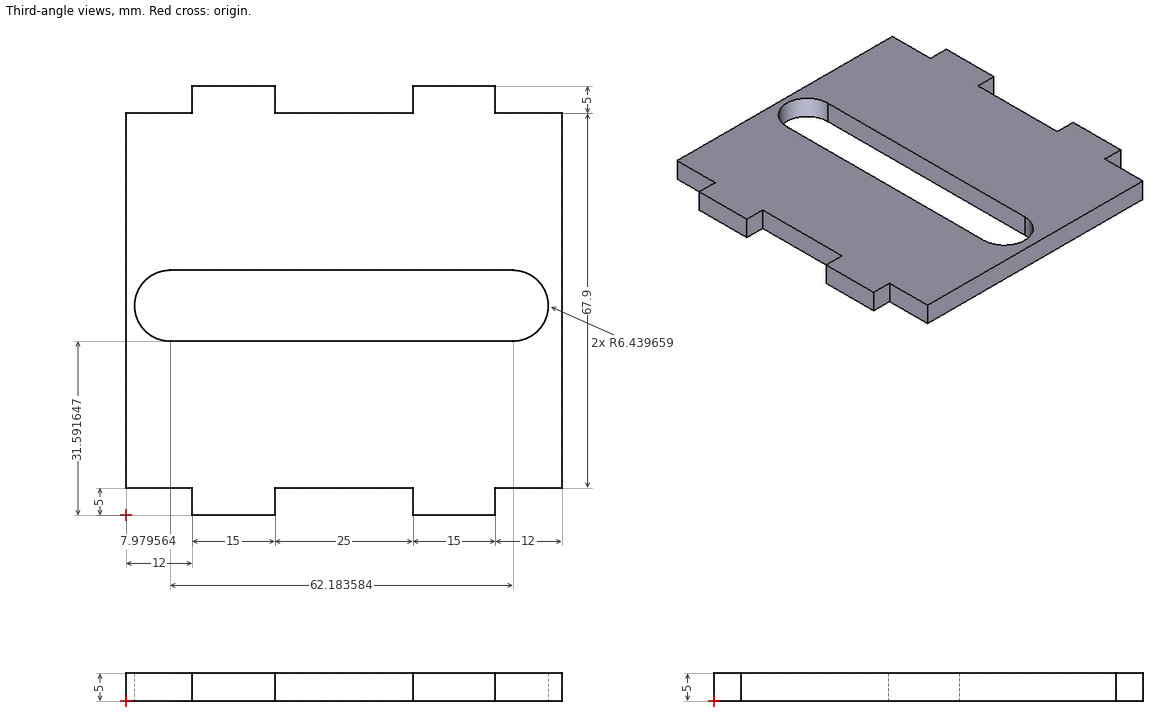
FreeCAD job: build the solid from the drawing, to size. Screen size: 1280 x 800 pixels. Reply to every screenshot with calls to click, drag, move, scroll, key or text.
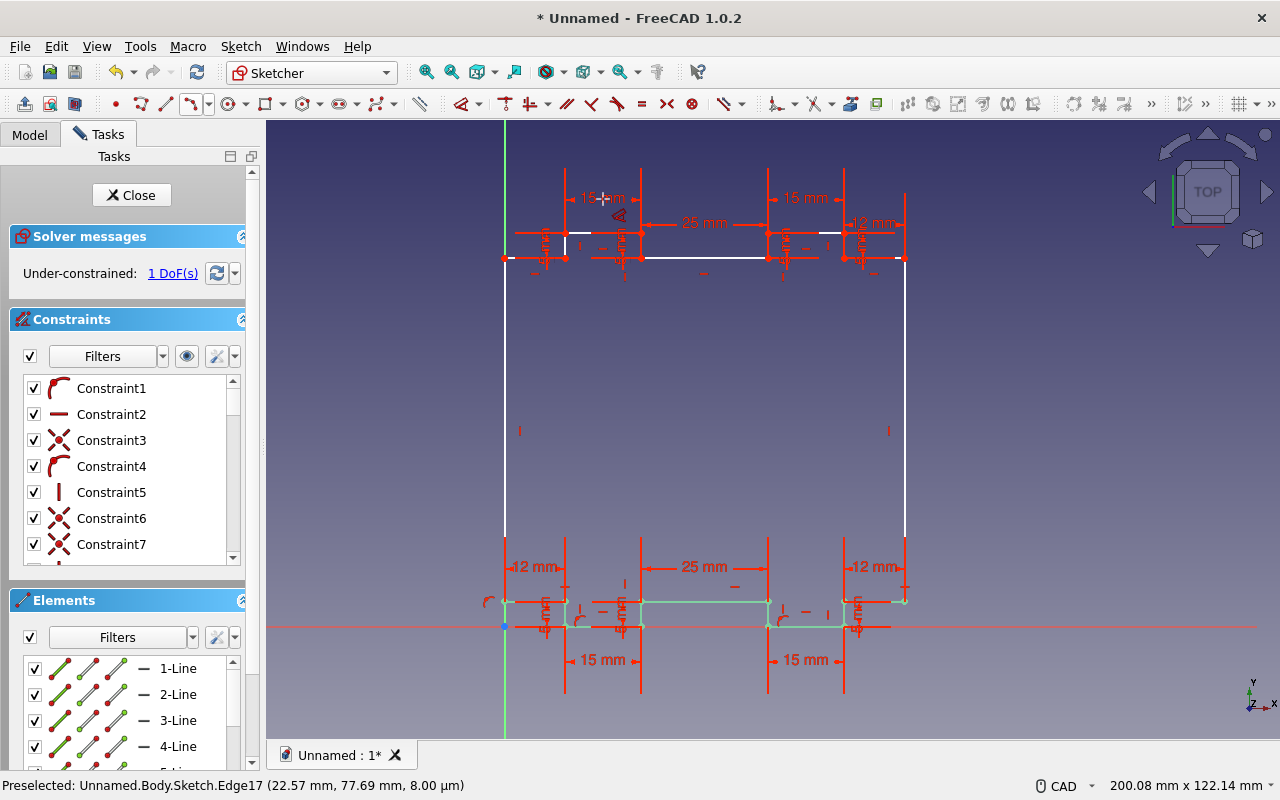
click(905, 499)
click(939, 430)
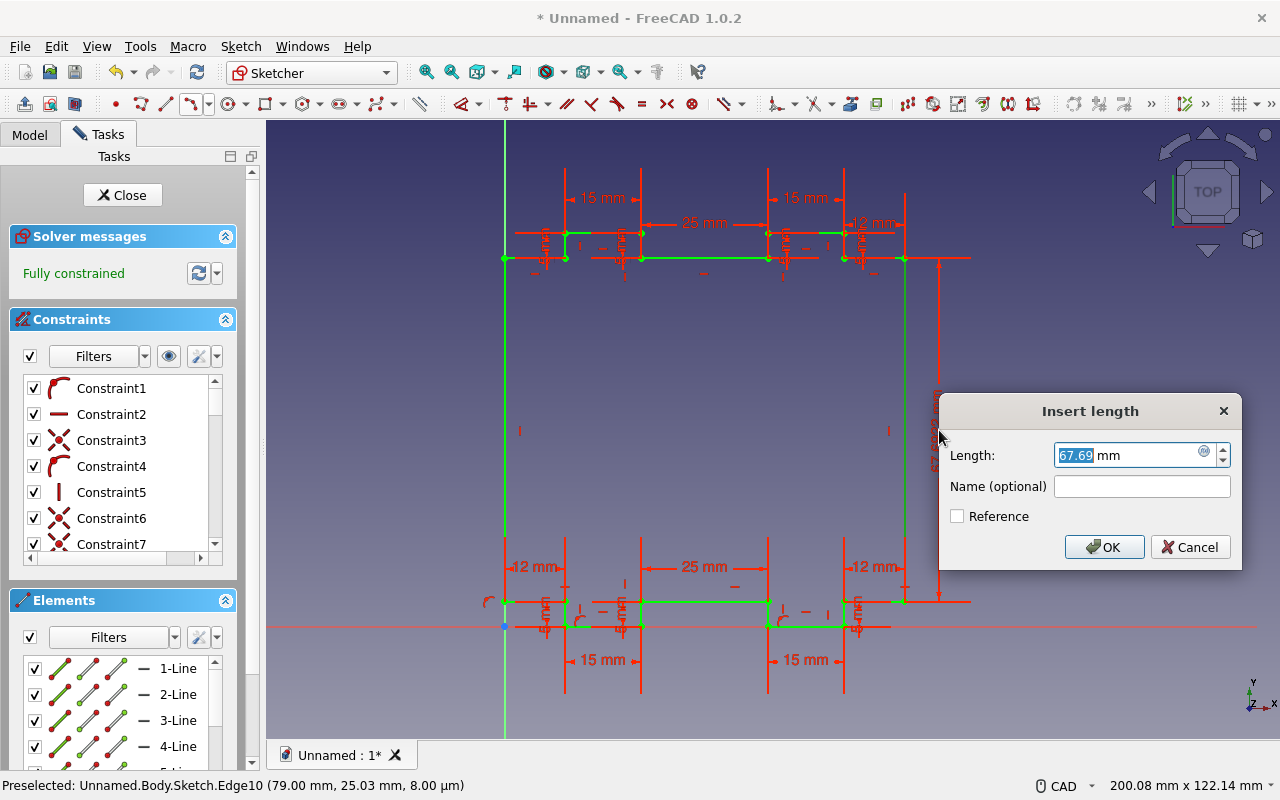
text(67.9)
key(Return)
key(Escape)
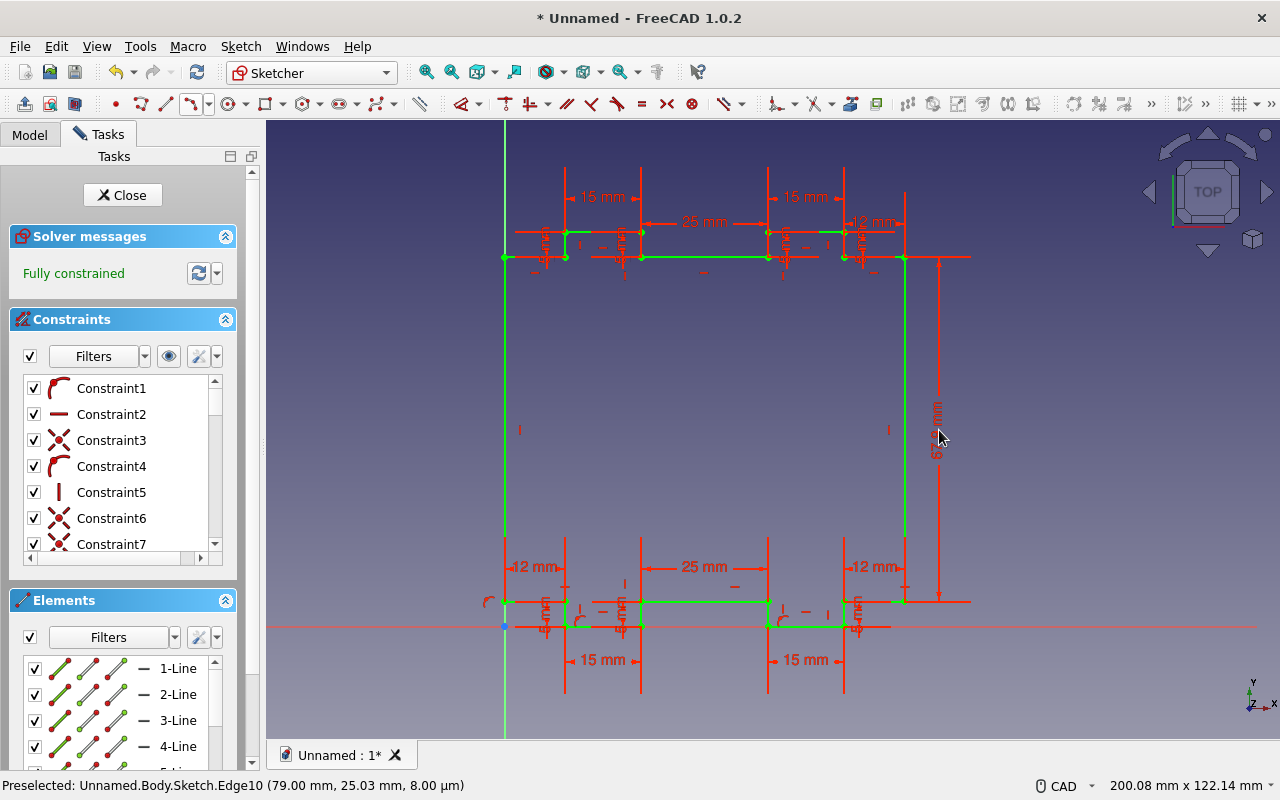
click(123, 195)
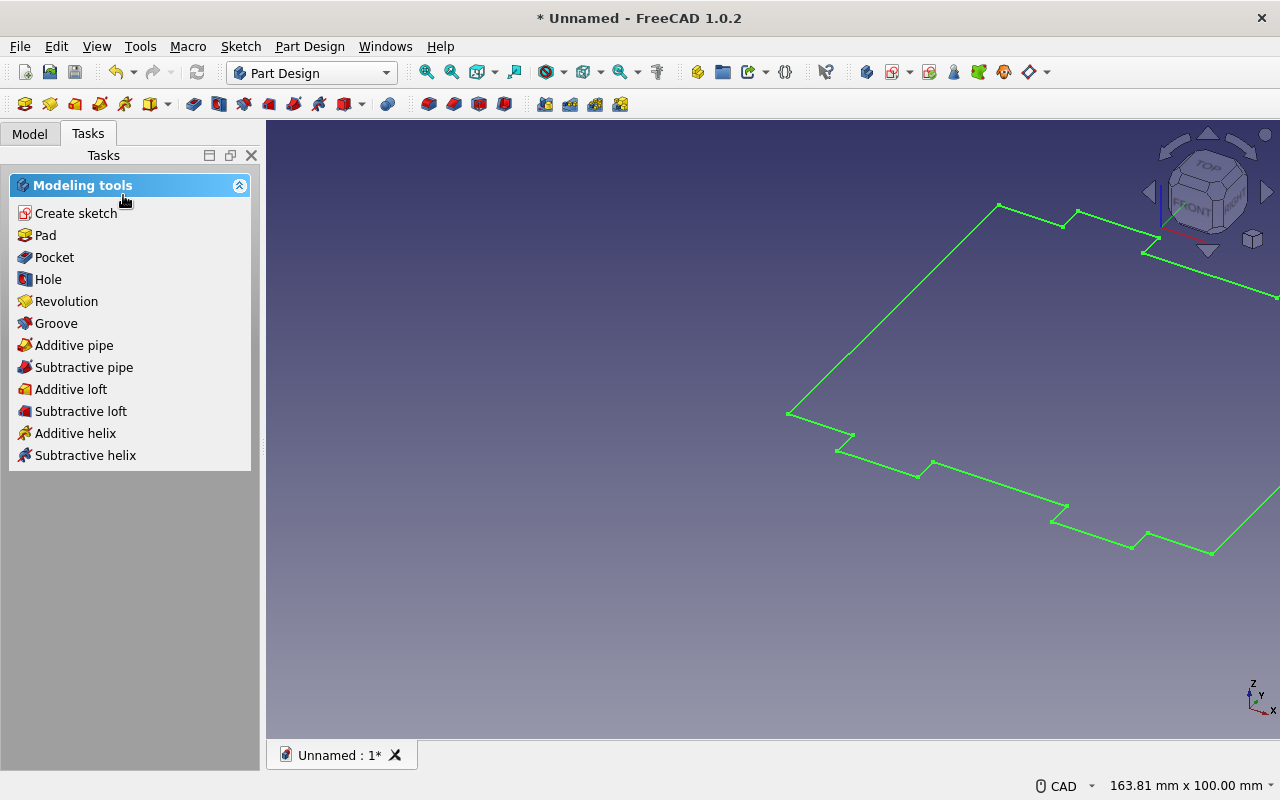
click(25, 104)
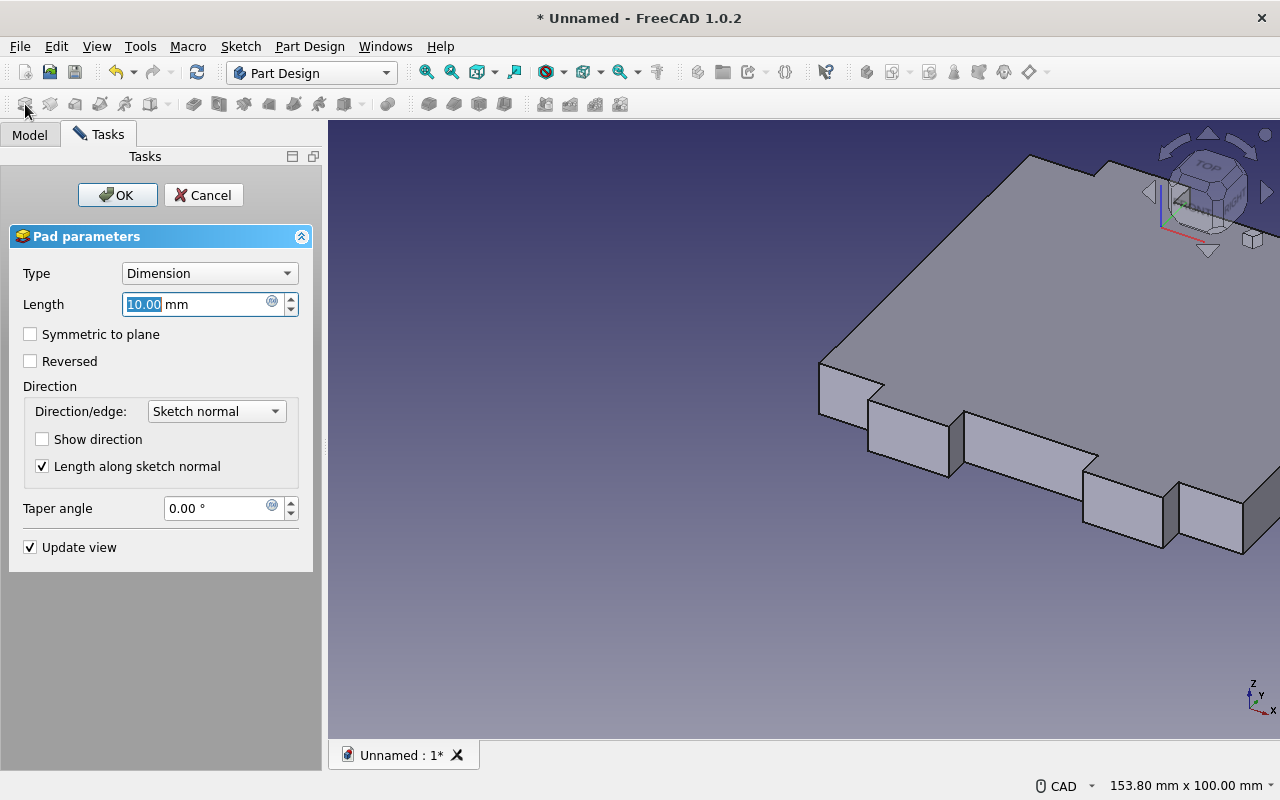
text(5)
key(Tab)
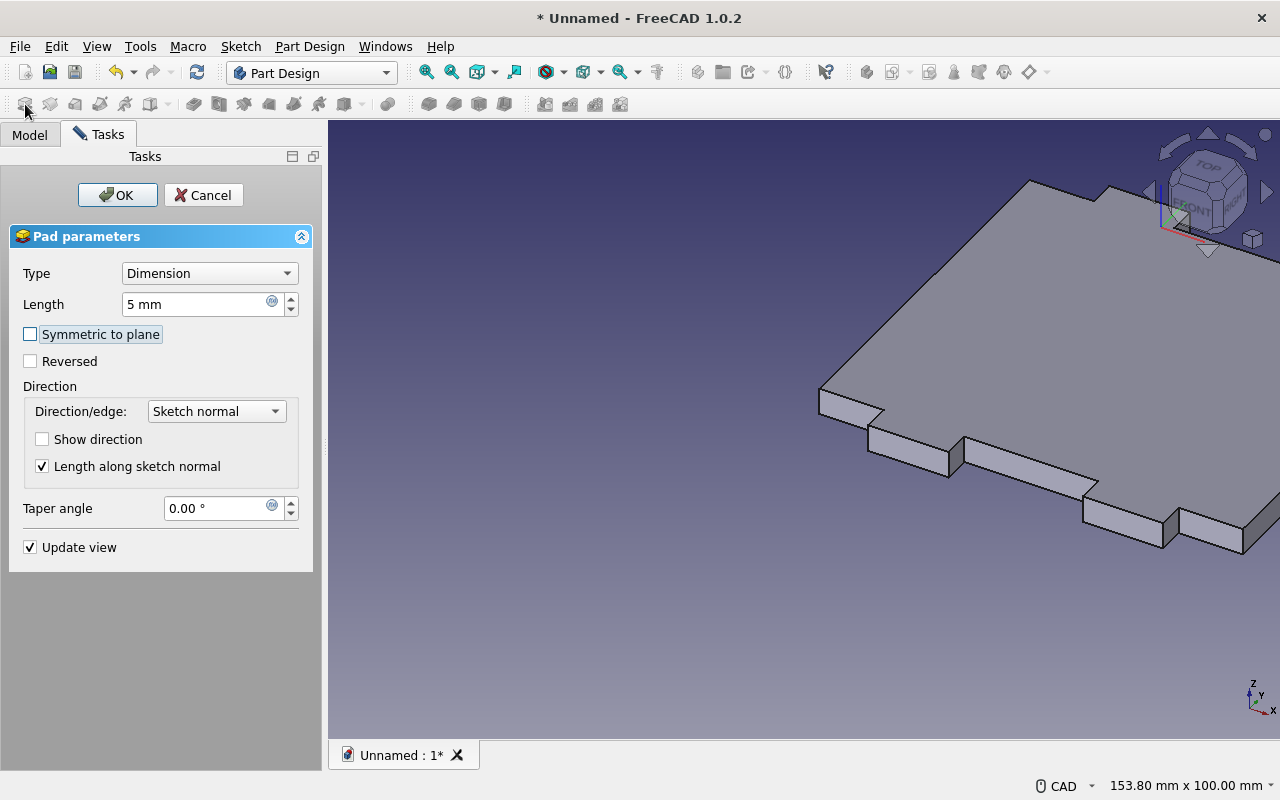
click(118, 195)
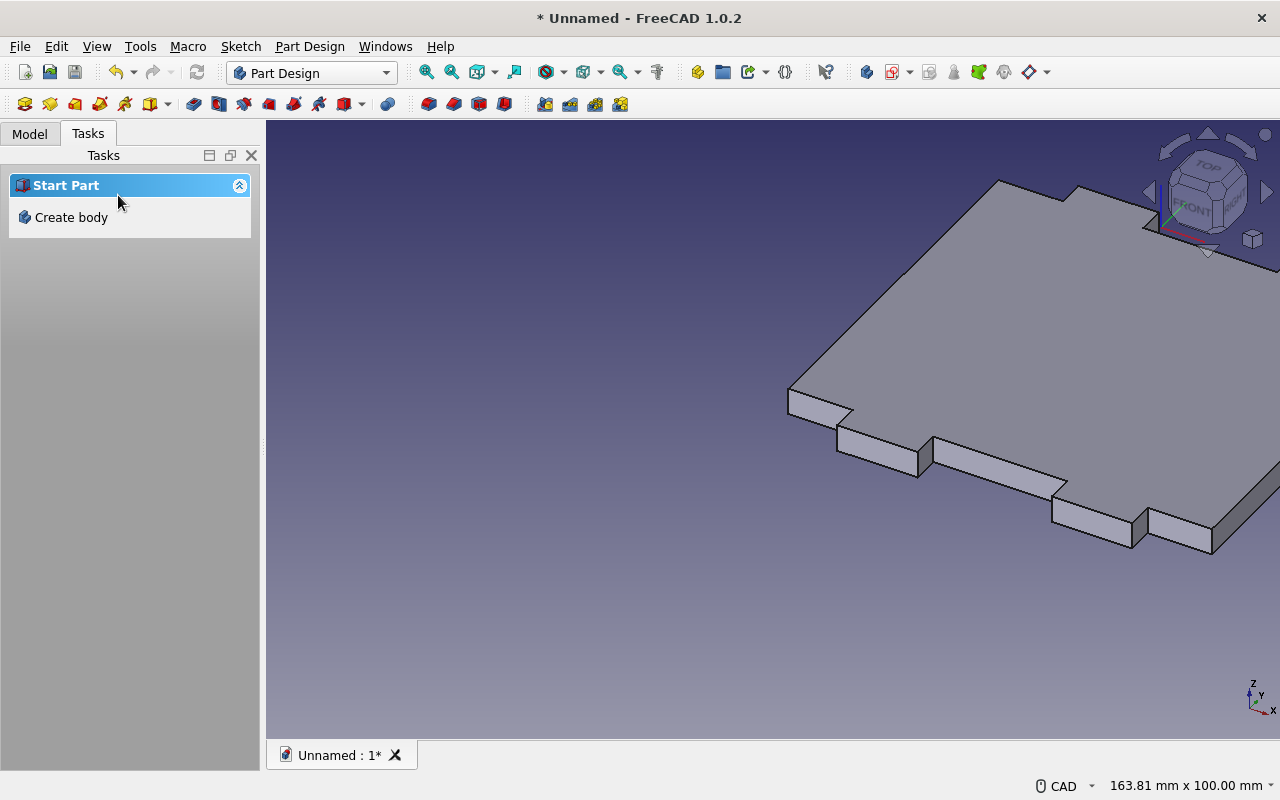
click(427, 72)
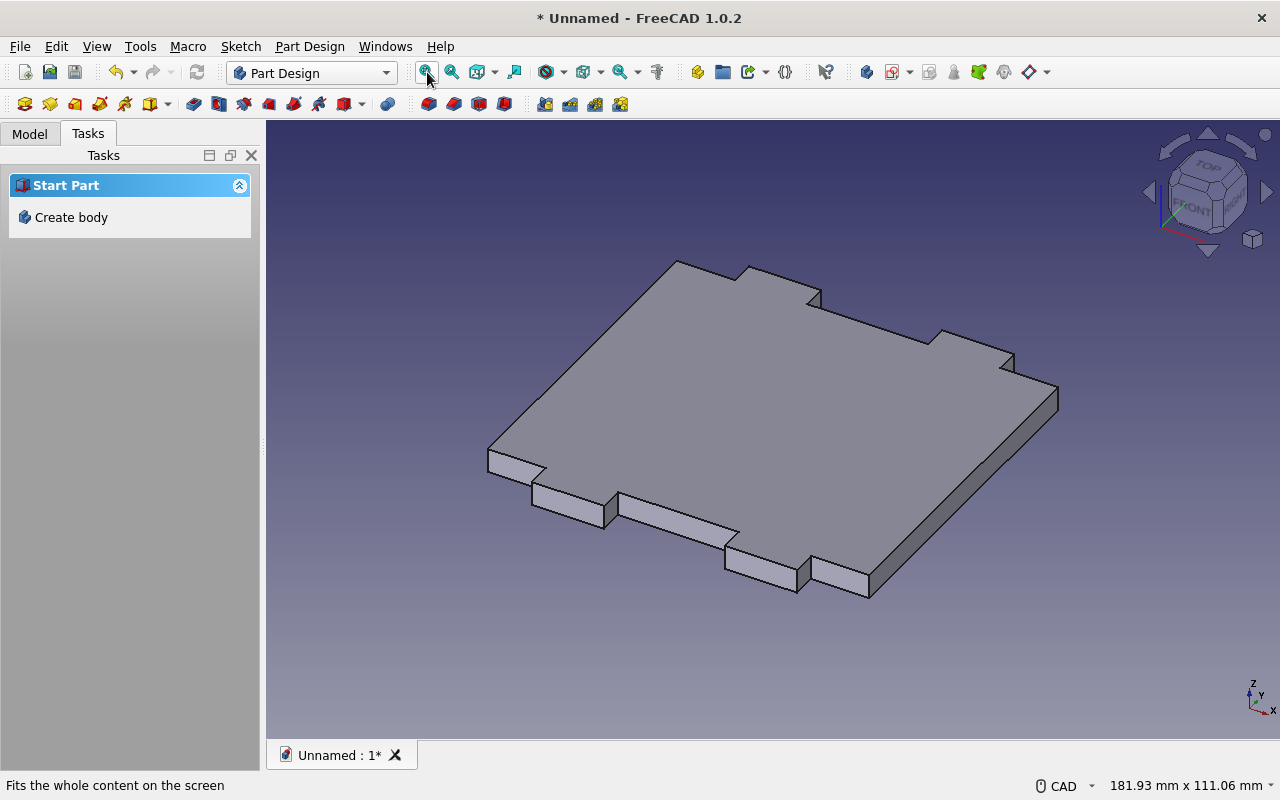
key(5)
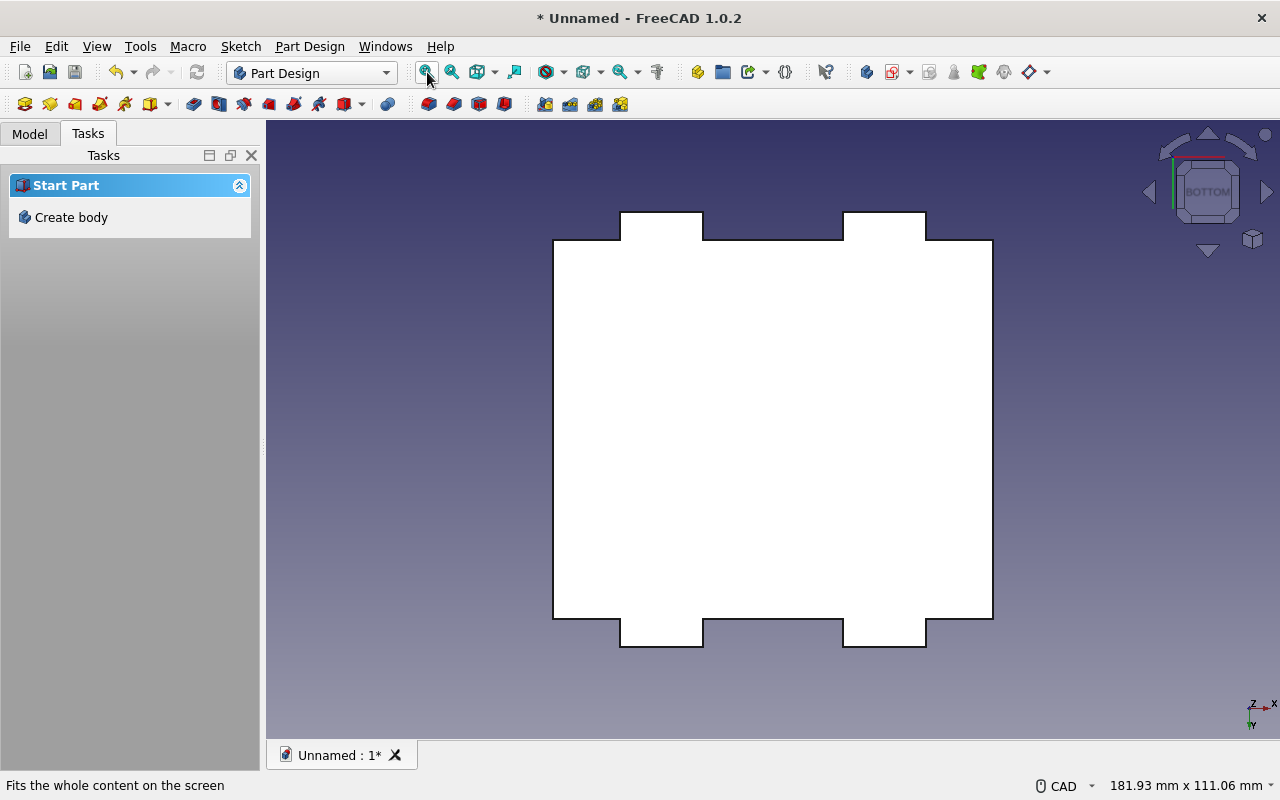
click(773, 428)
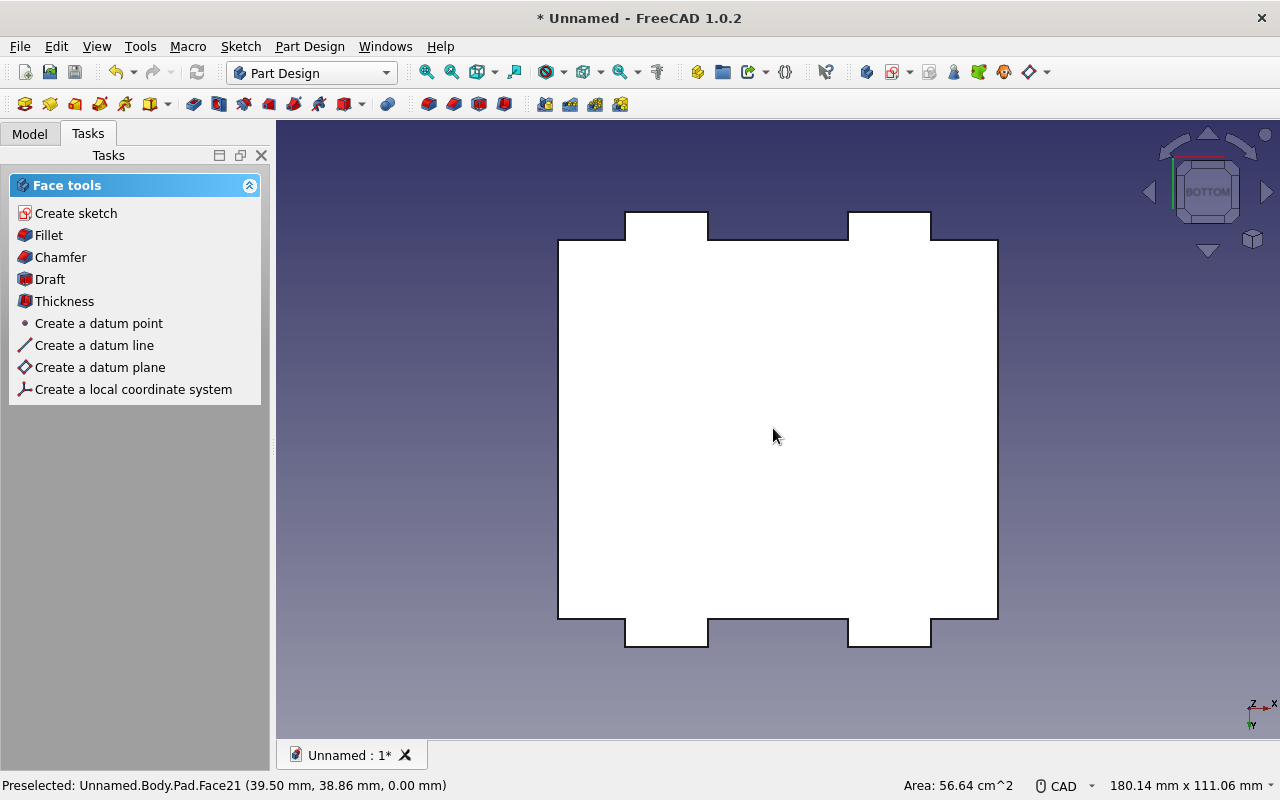
click(892, 72)